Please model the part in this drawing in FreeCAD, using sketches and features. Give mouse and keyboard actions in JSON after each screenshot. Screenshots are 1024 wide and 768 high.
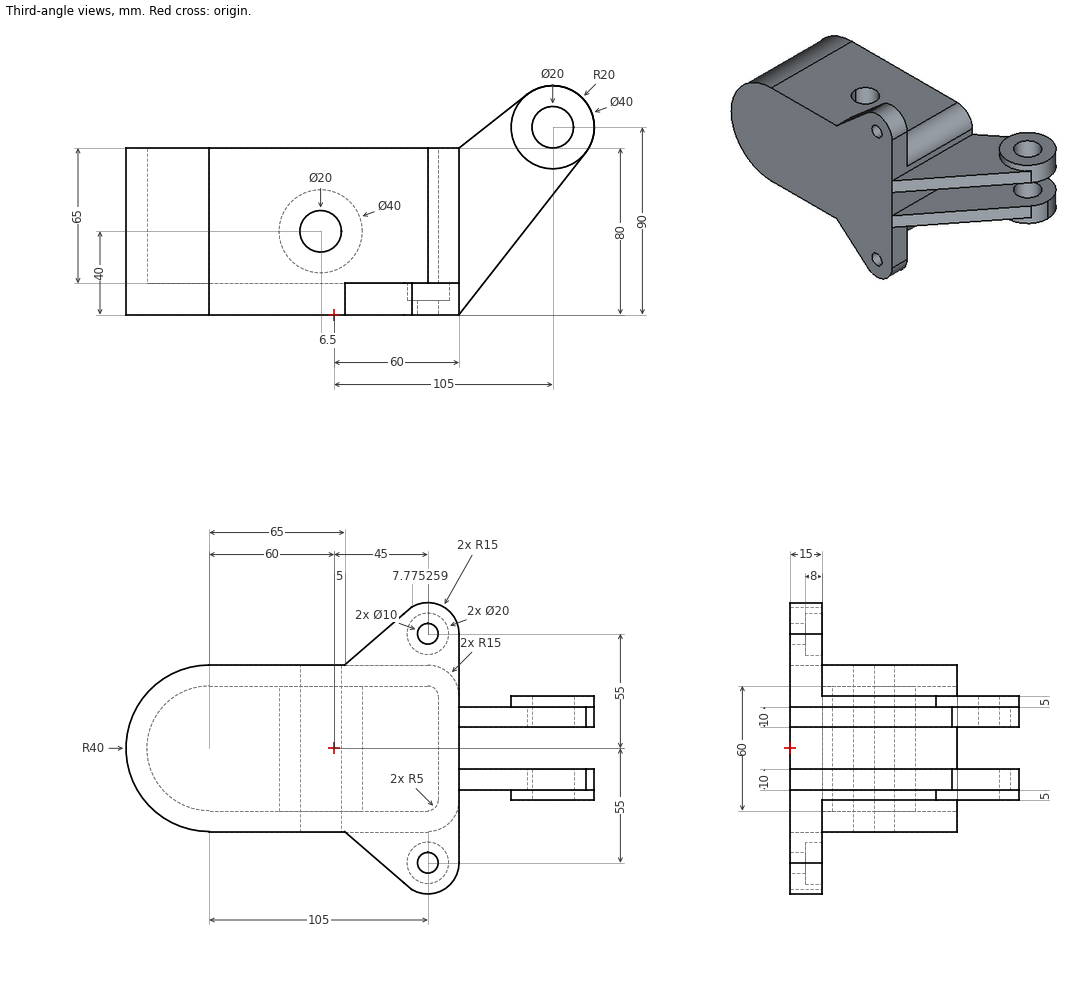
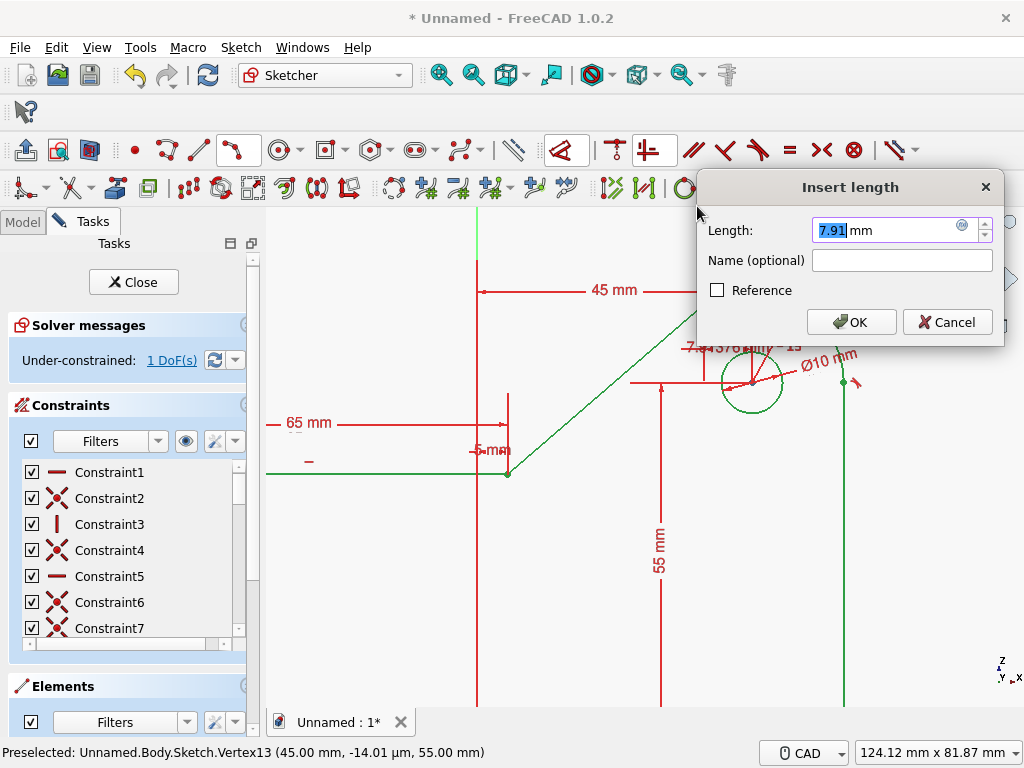
{"action": "type", "text": "7.775259"}
{"action": "key", "text": "Return"}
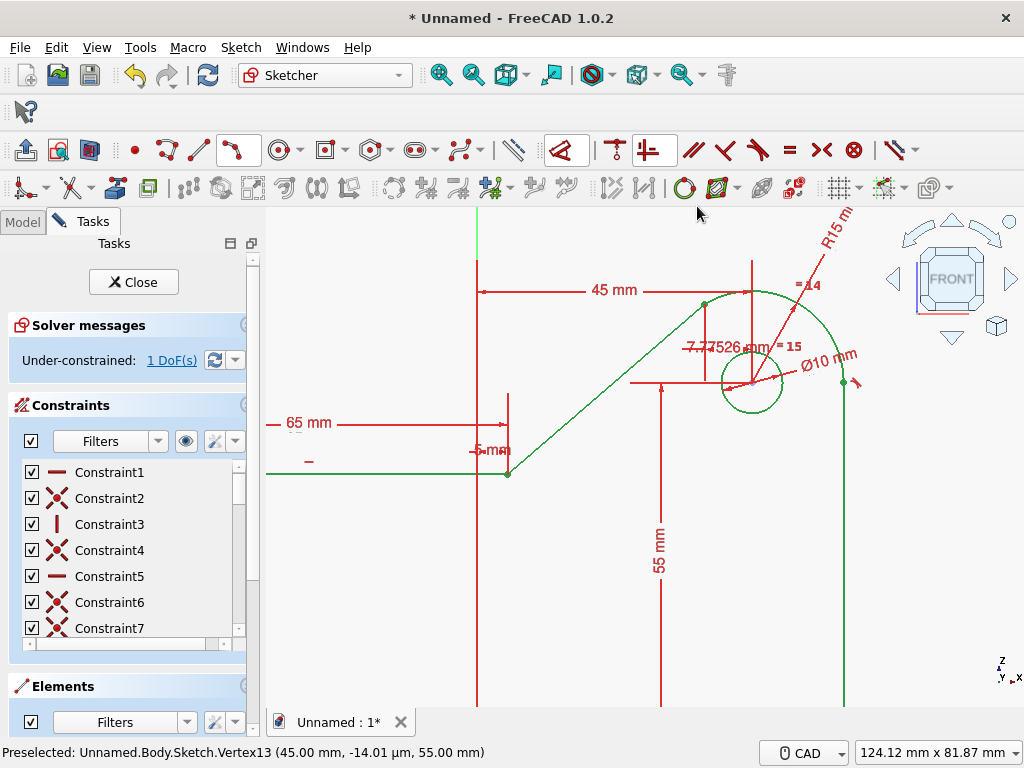
{"action": "scroll", "coordinate": [705, 305], "scroll_direction": "down", "scroll_amount": 5}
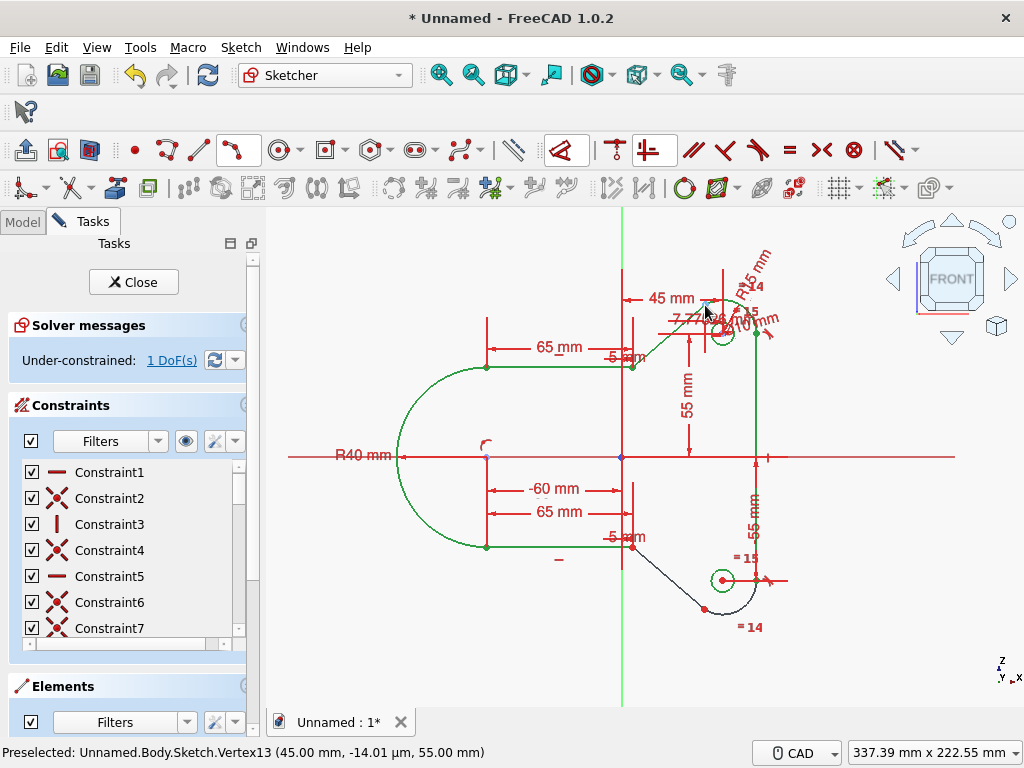
{"action": "scroll", "coordinate": [705, 610], "scroll_direction": "up", "scroll_amount": 5}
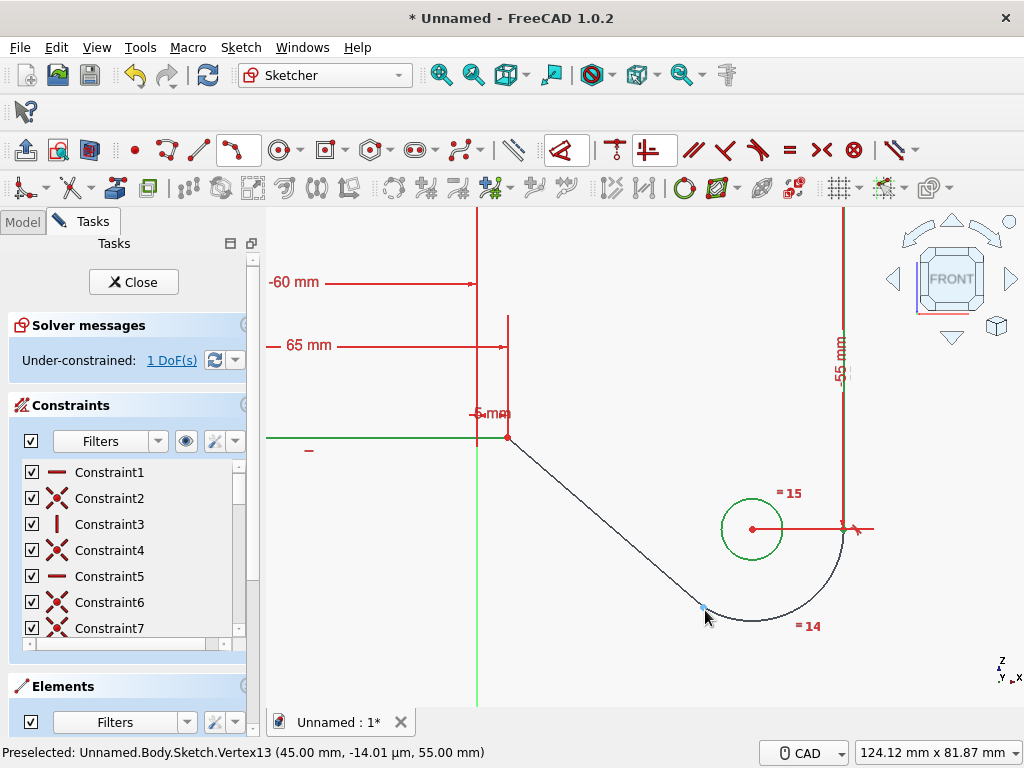
{"action": "left_click", "coordinate": [704, 607]}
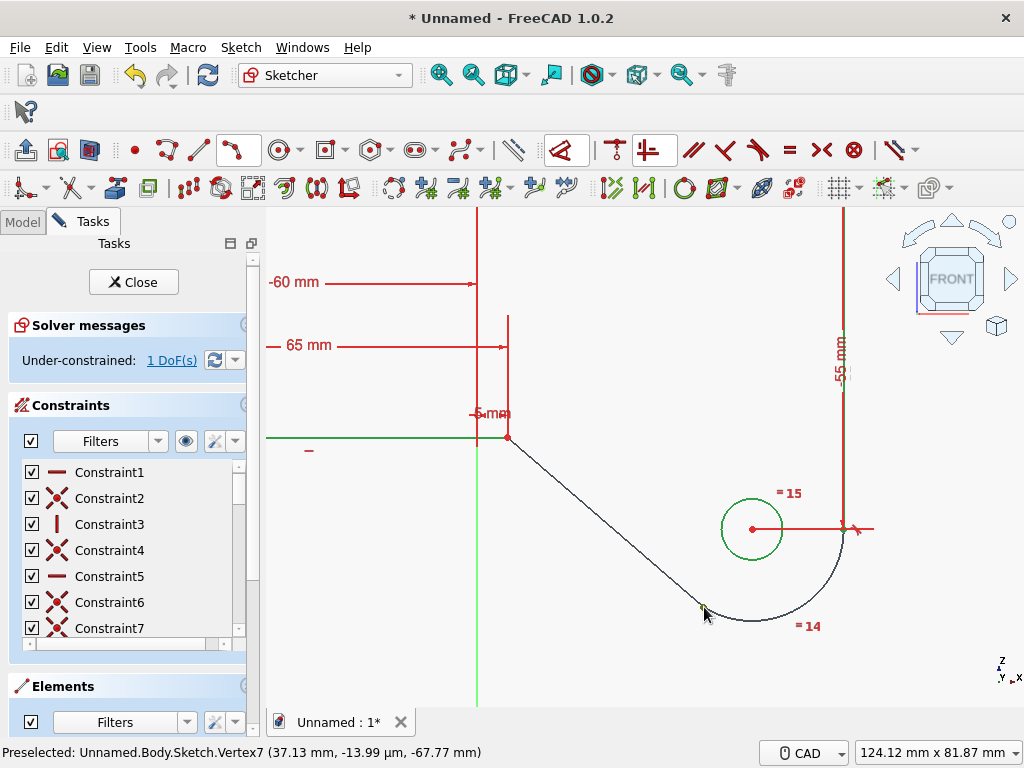
{"action": "left_click", "coordinate": [752, 529]}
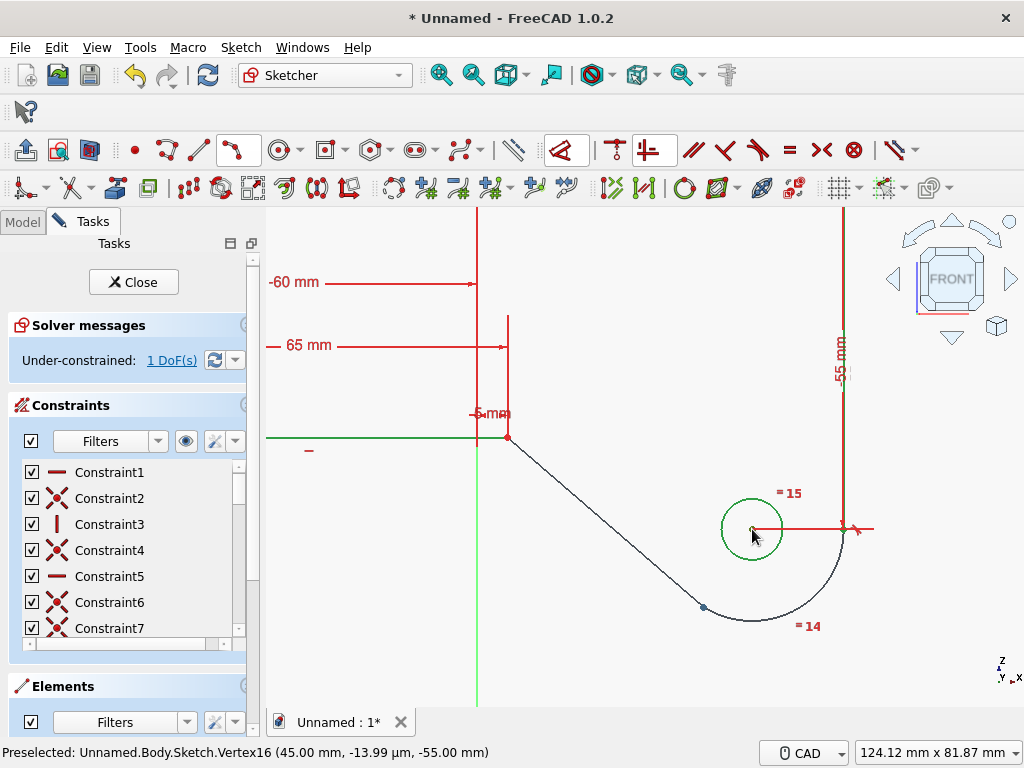
{"action": "left_click", "coordinate": [584, 150]}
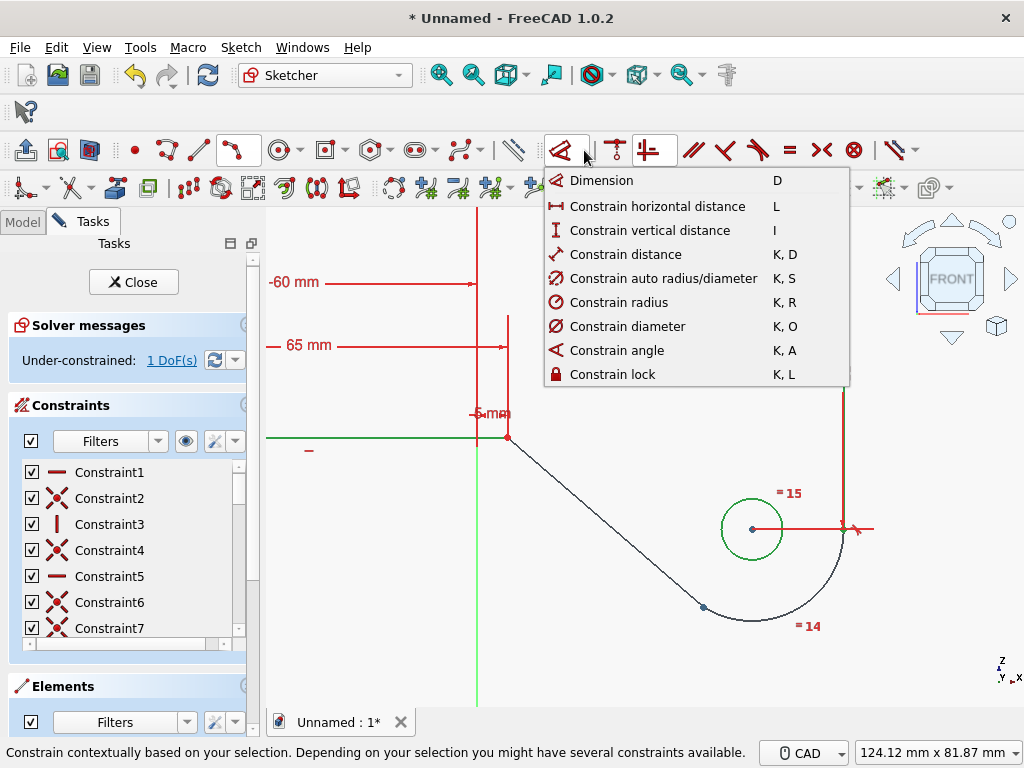
{"action": "left_click", "coordinate": [697, 206]}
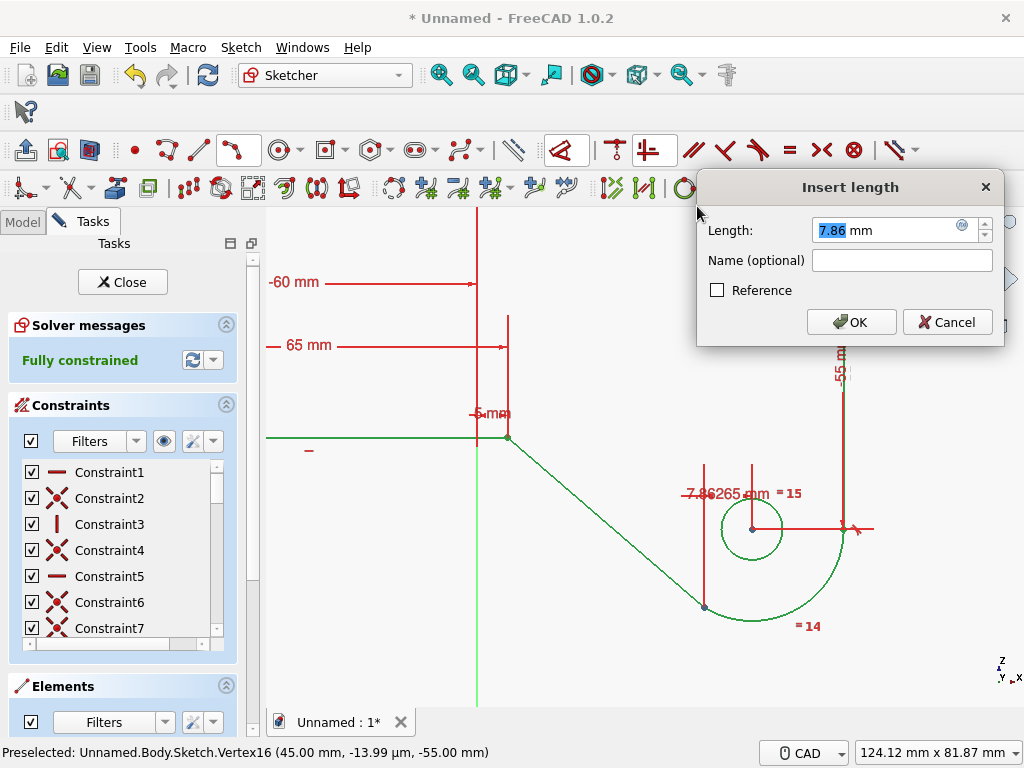
{"action": "type", "text": "7.775259"}
{"action": "key", "text": "Return"}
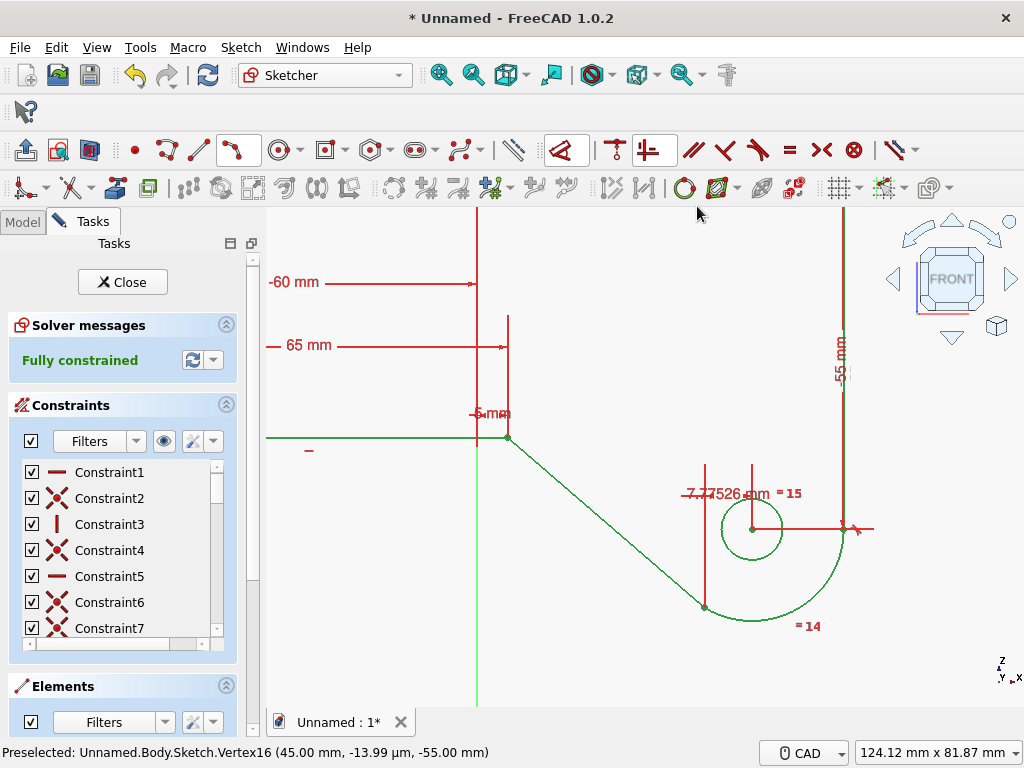
{"action": "left_click", "coordinate": [123, 282]}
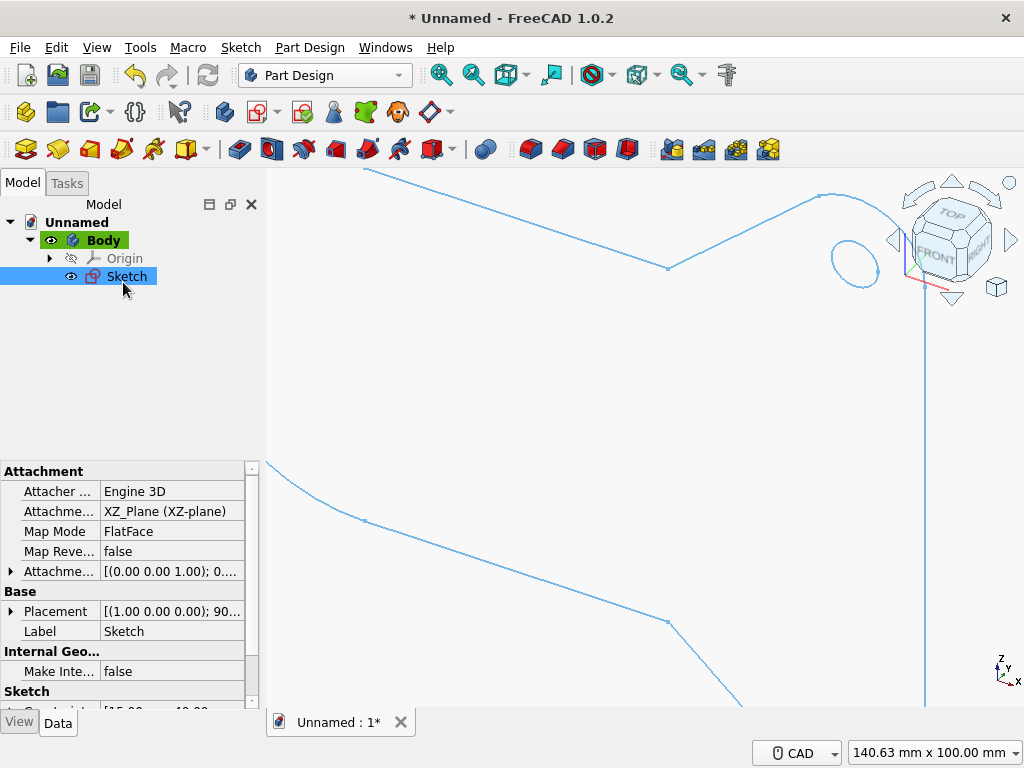
{"action": "left_click", "coordinate": [26, 150]}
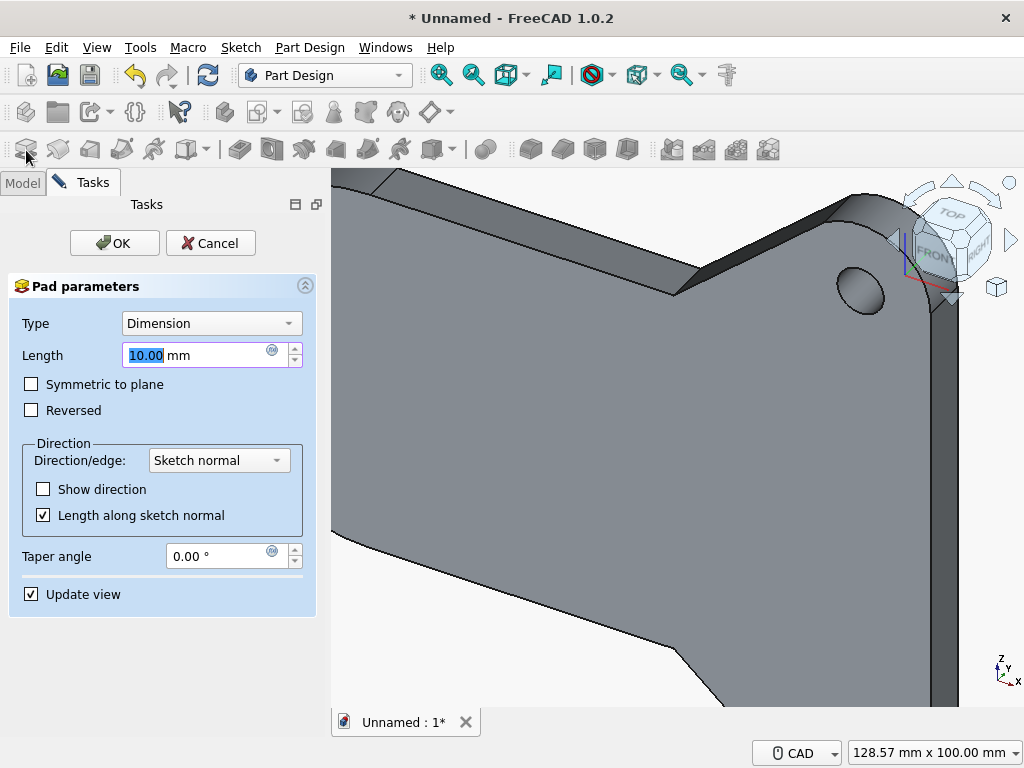
{"action": "type", "text": "15"}
{"action": "key", "text": "Tab"}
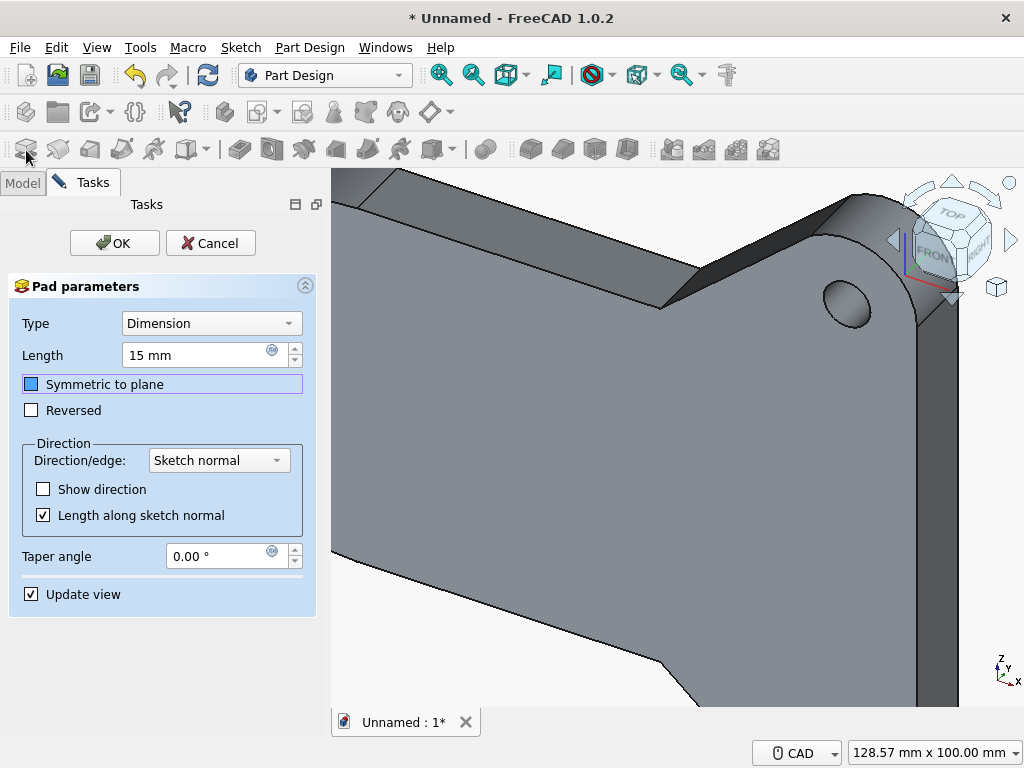
{"action": "left_click", "coordinate": [30, 410]}